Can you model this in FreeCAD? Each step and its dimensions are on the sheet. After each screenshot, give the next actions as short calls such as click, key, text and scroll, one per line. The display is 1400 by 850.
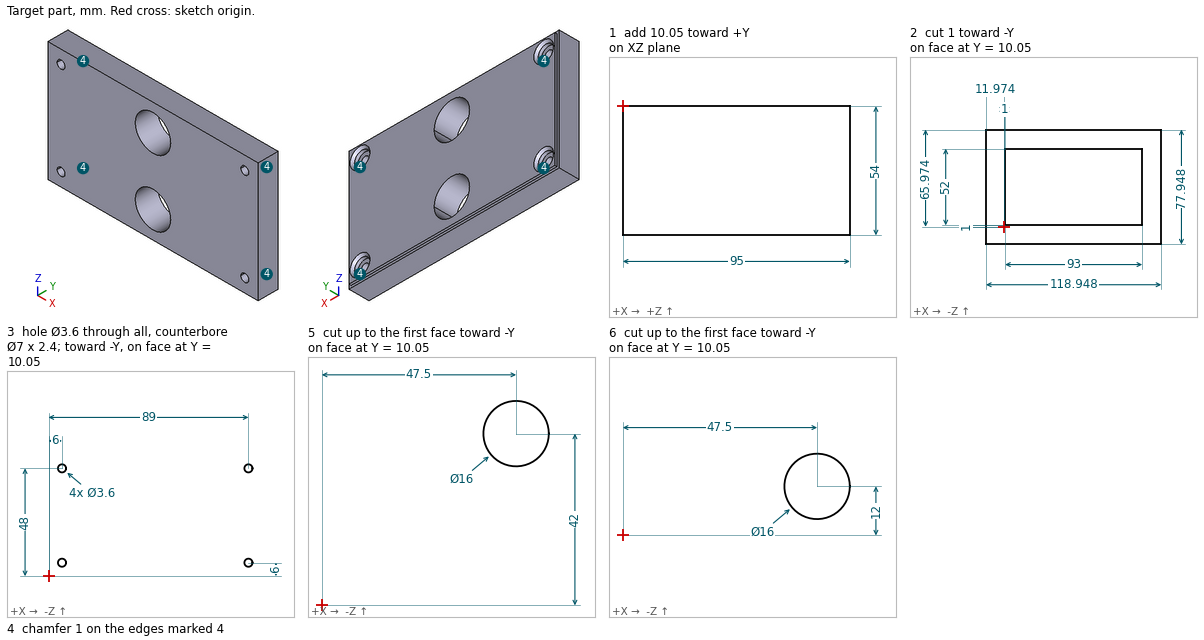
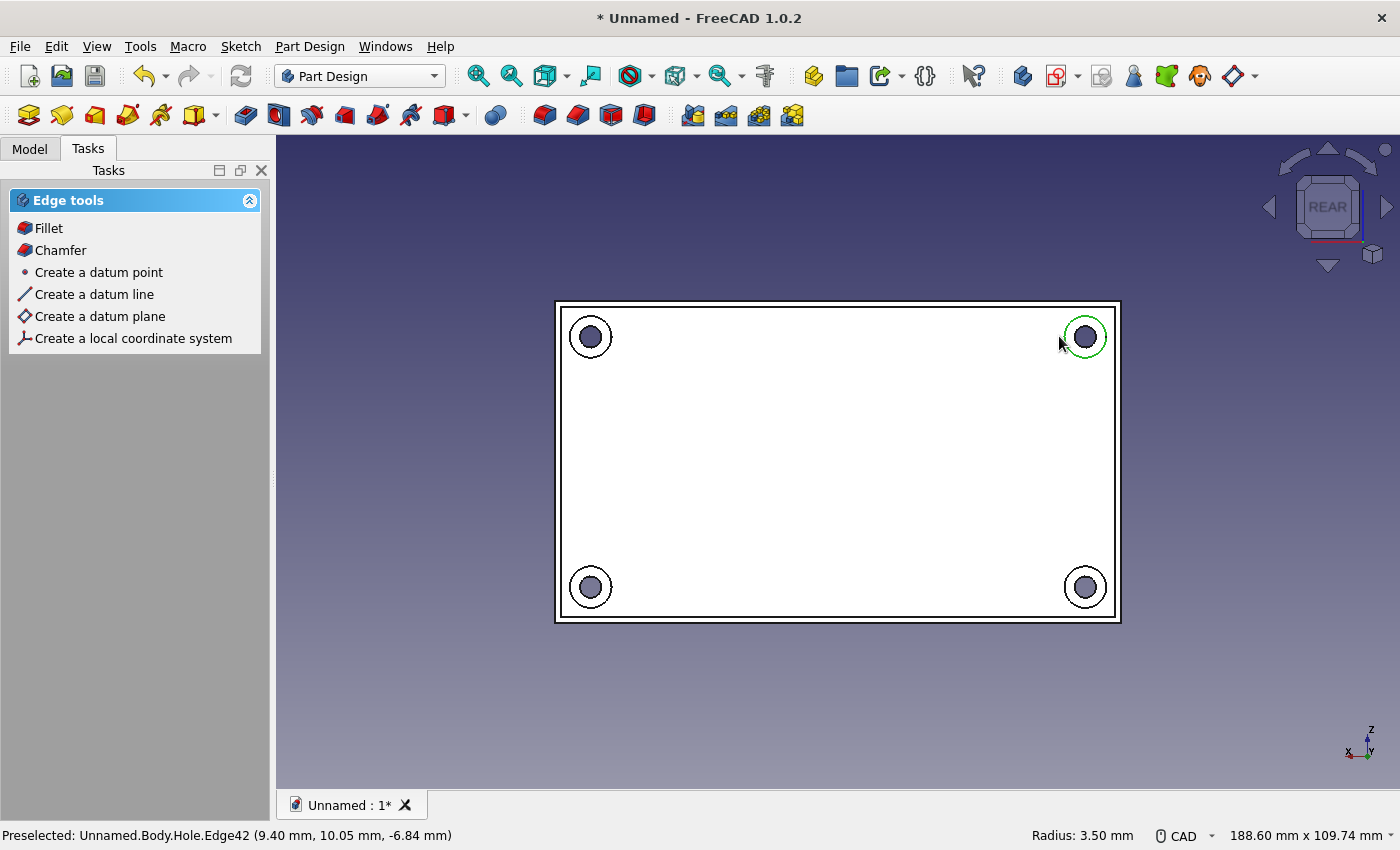
click(570, 336, ctrl)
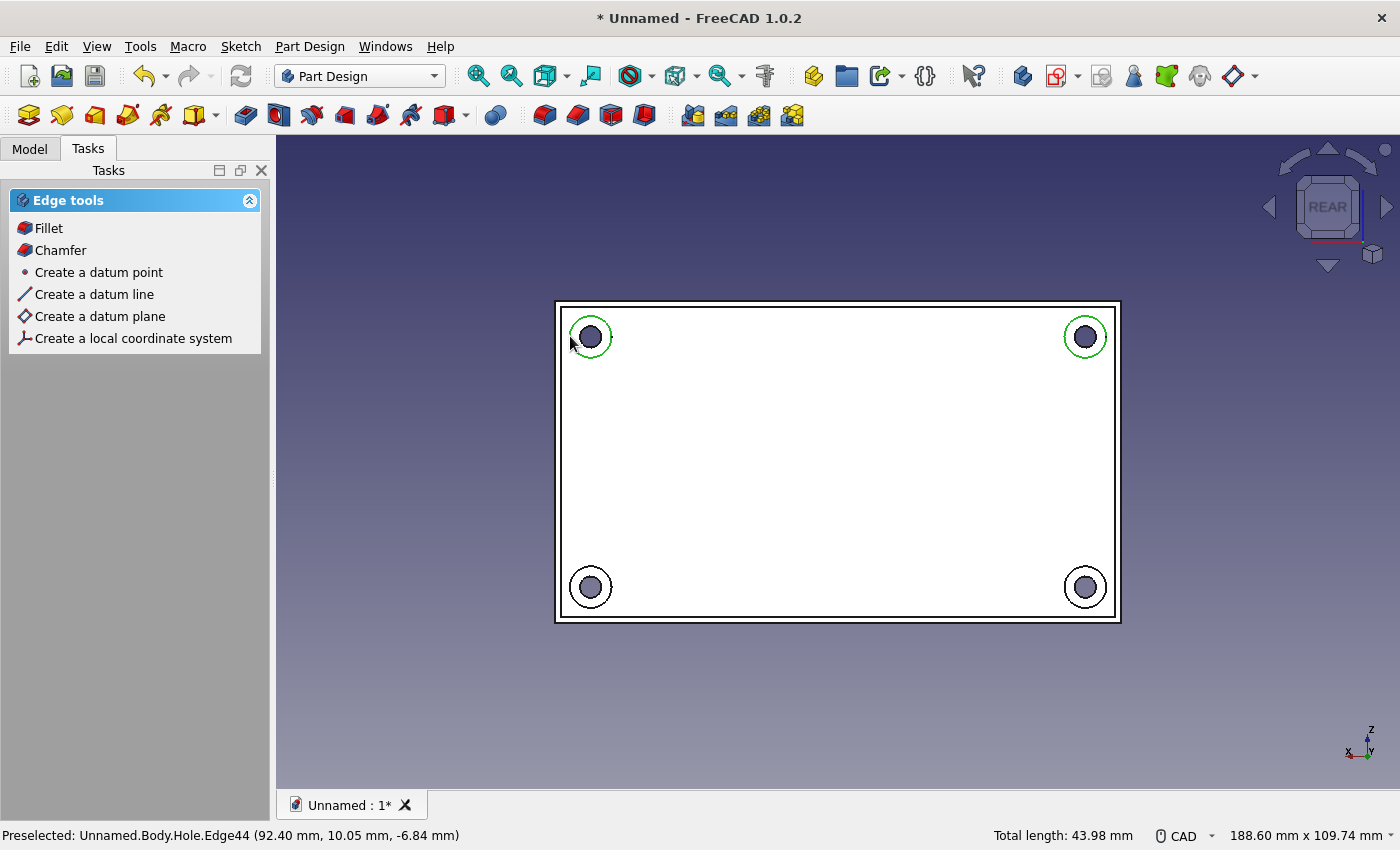
click(570, 586, ctrl)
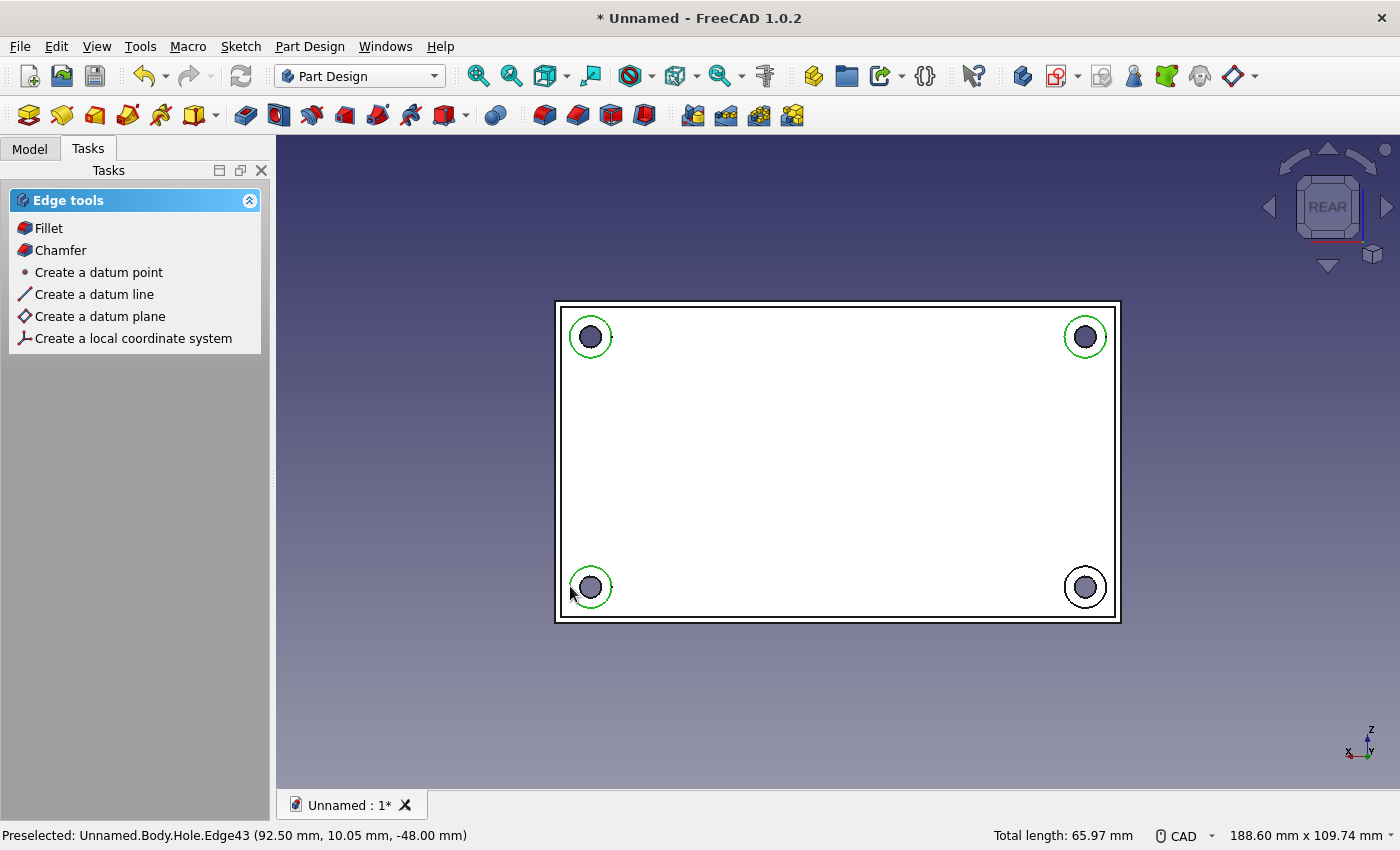
click(1064, 586, ctrl)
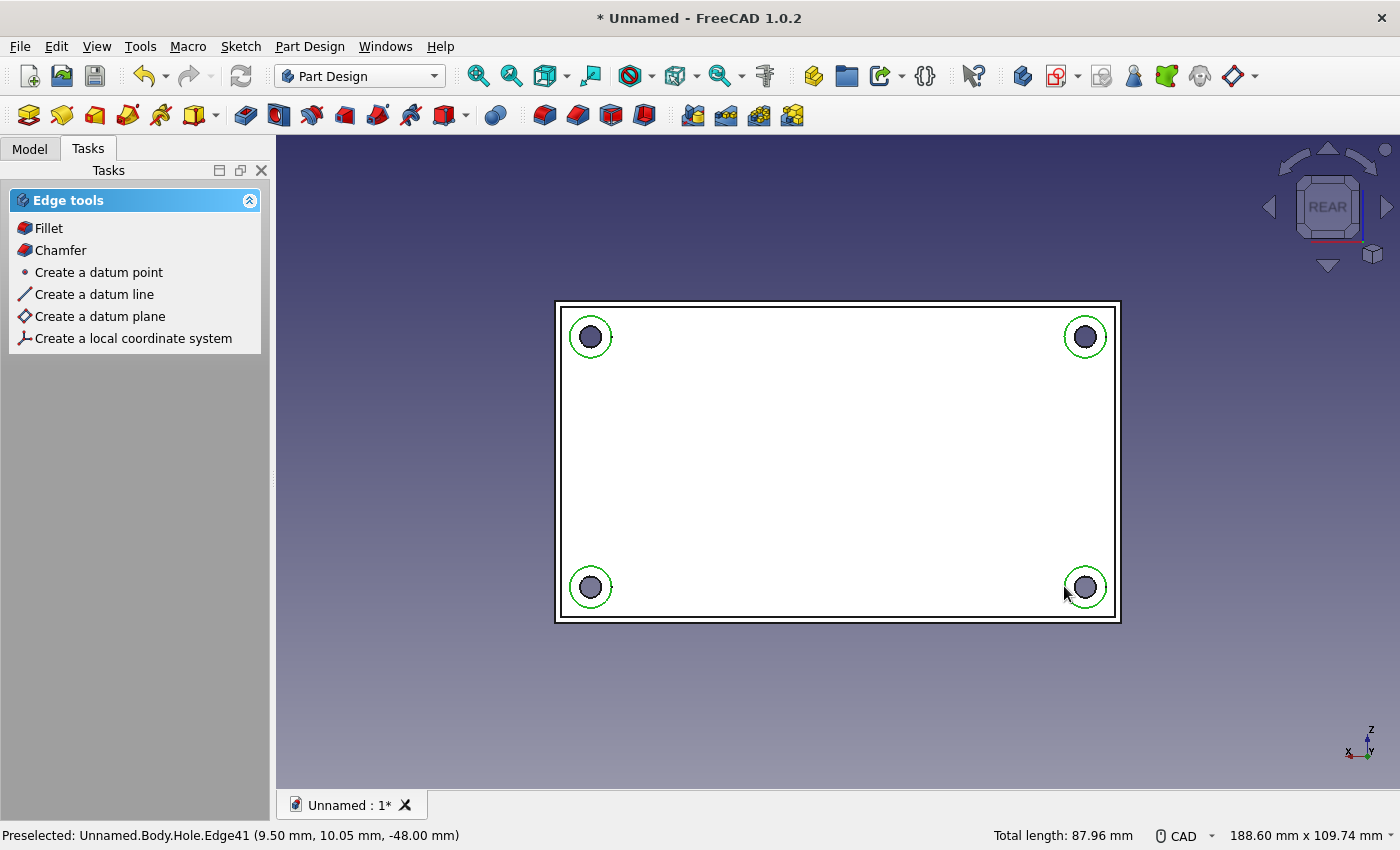
click(578, 116)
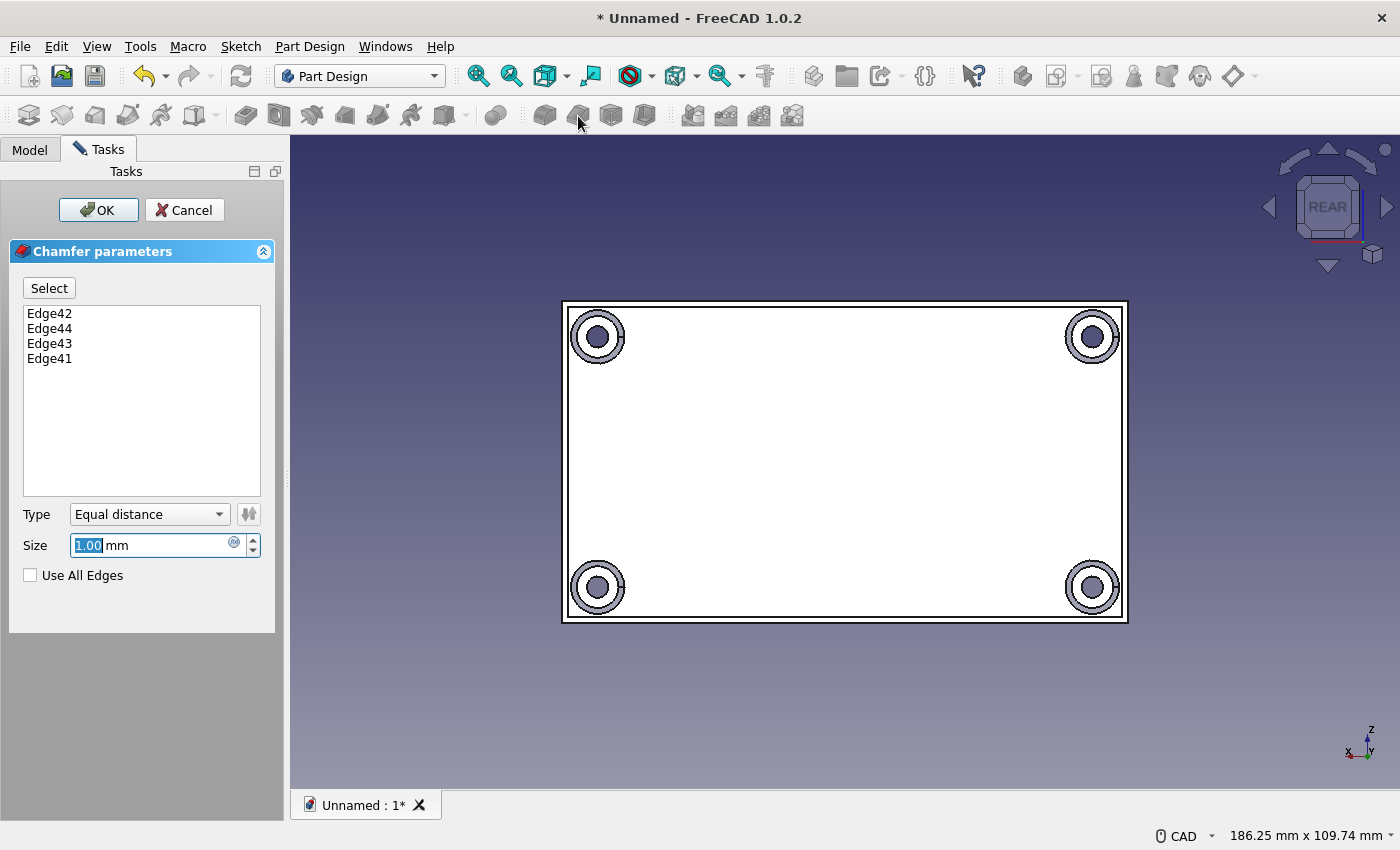
text(1)
key(Tab)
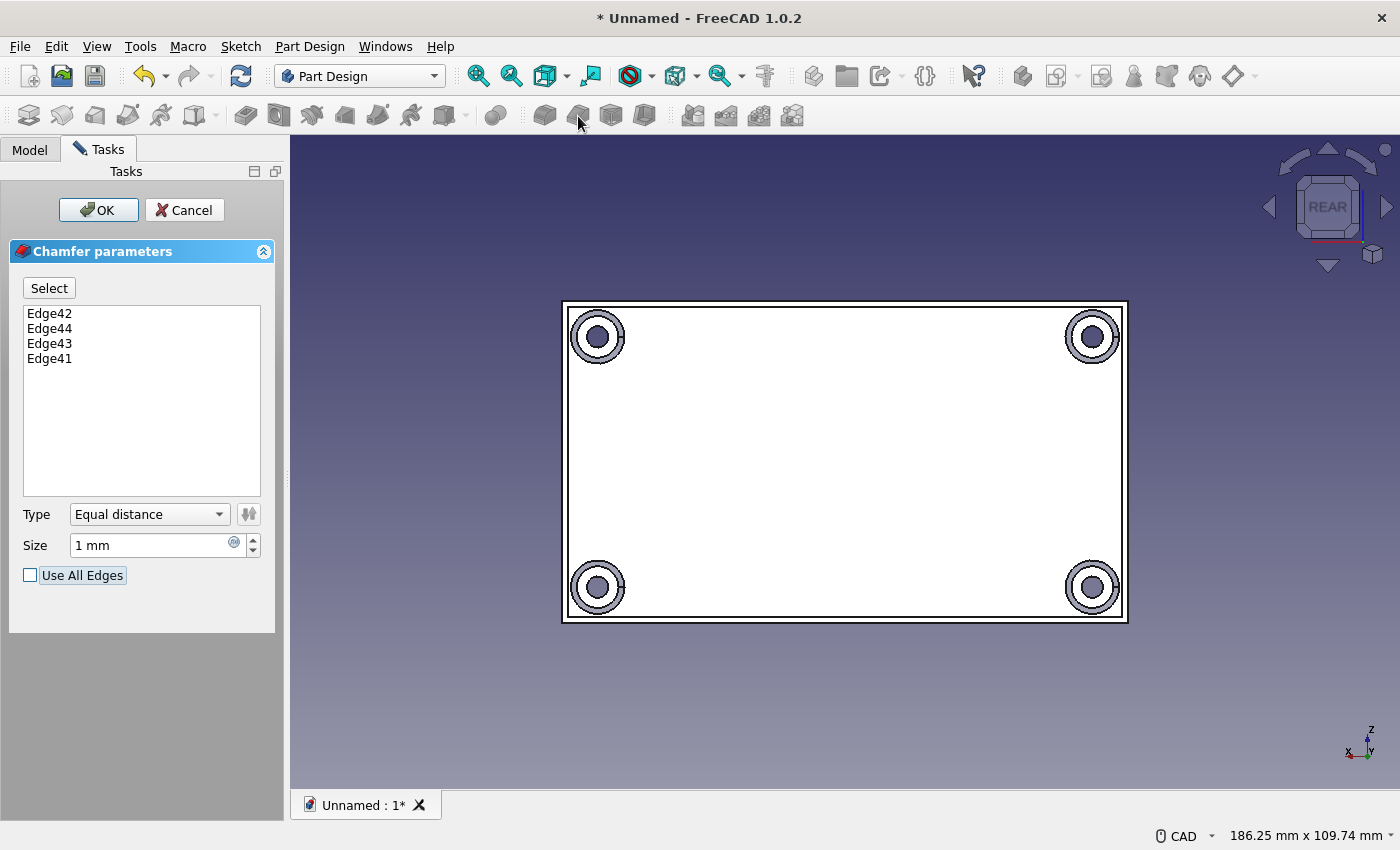
click(99, 210)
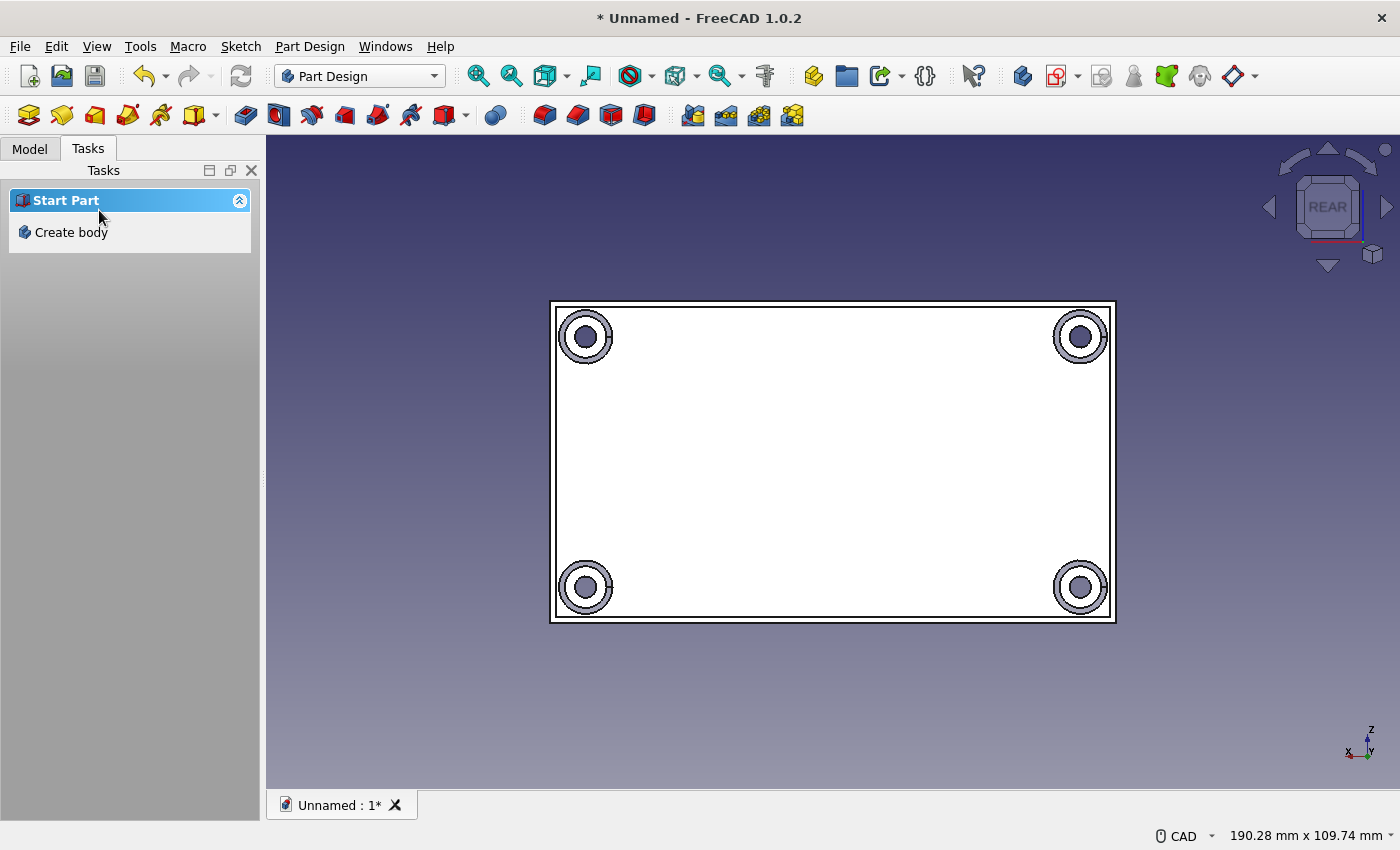
click(754, 461)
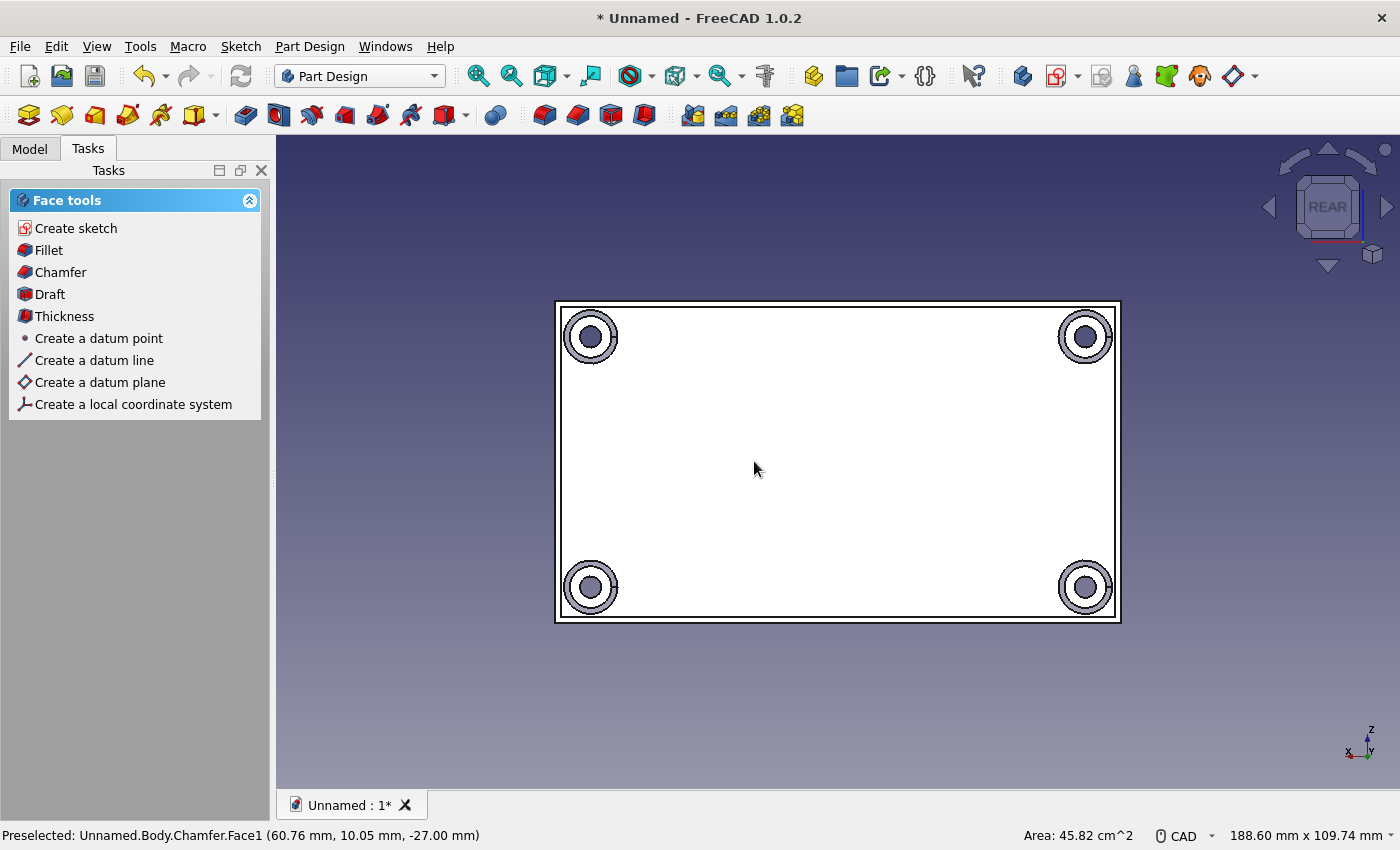
click(1056, 76)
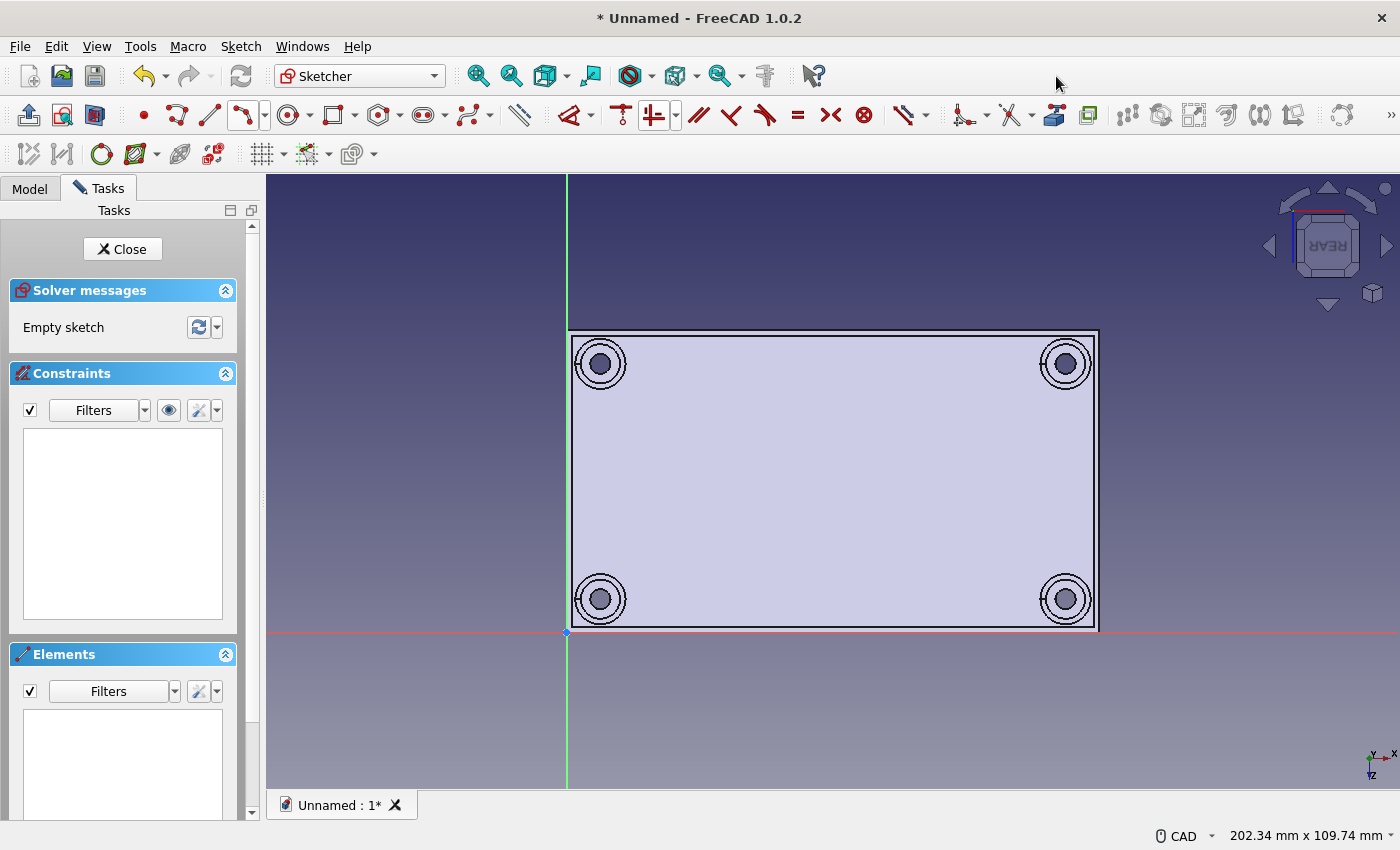
scroll(855, 370, up, 7)